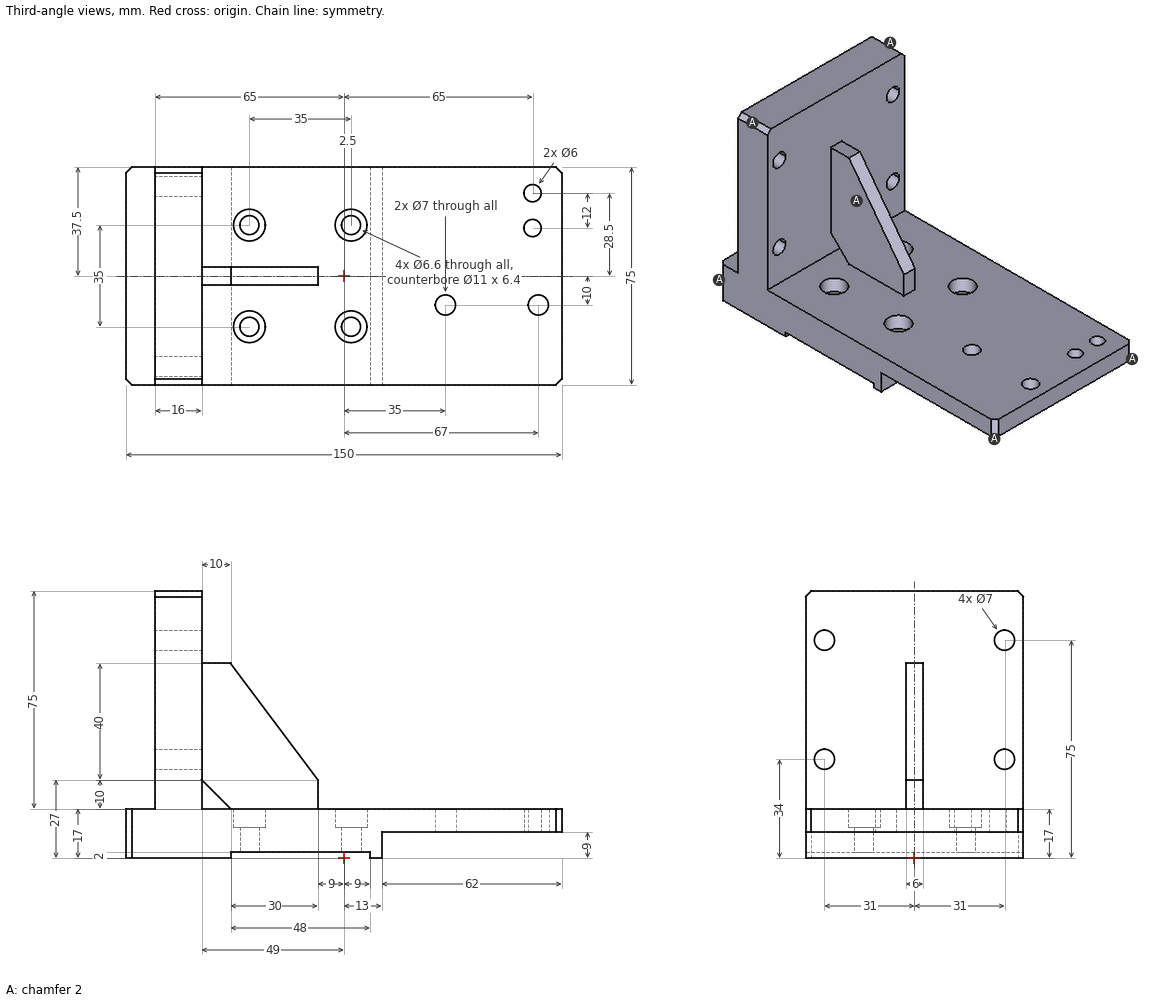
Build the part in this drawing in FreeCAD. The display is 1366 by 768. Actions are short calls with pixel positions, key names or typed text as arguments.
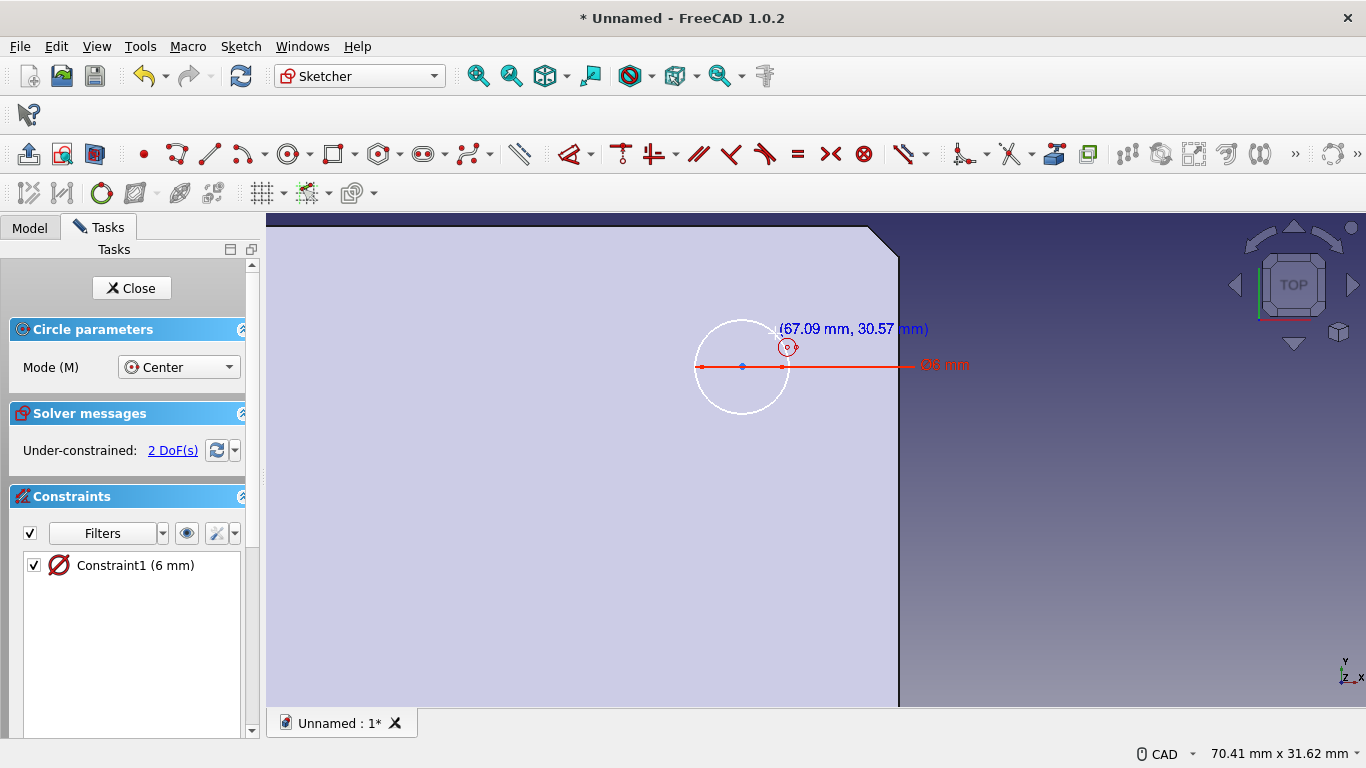
click(742, 554)
move(775, 521)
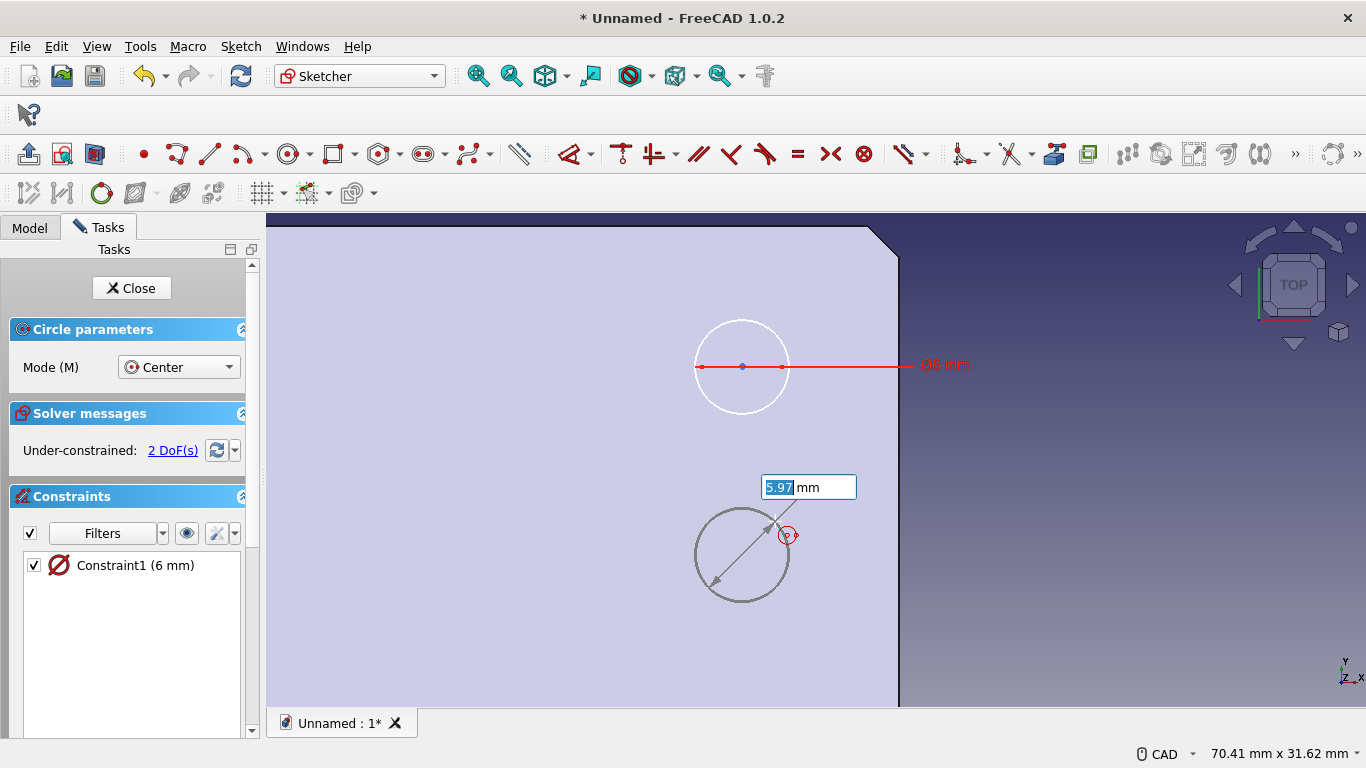
text(6)
key(Return)
key(Escape)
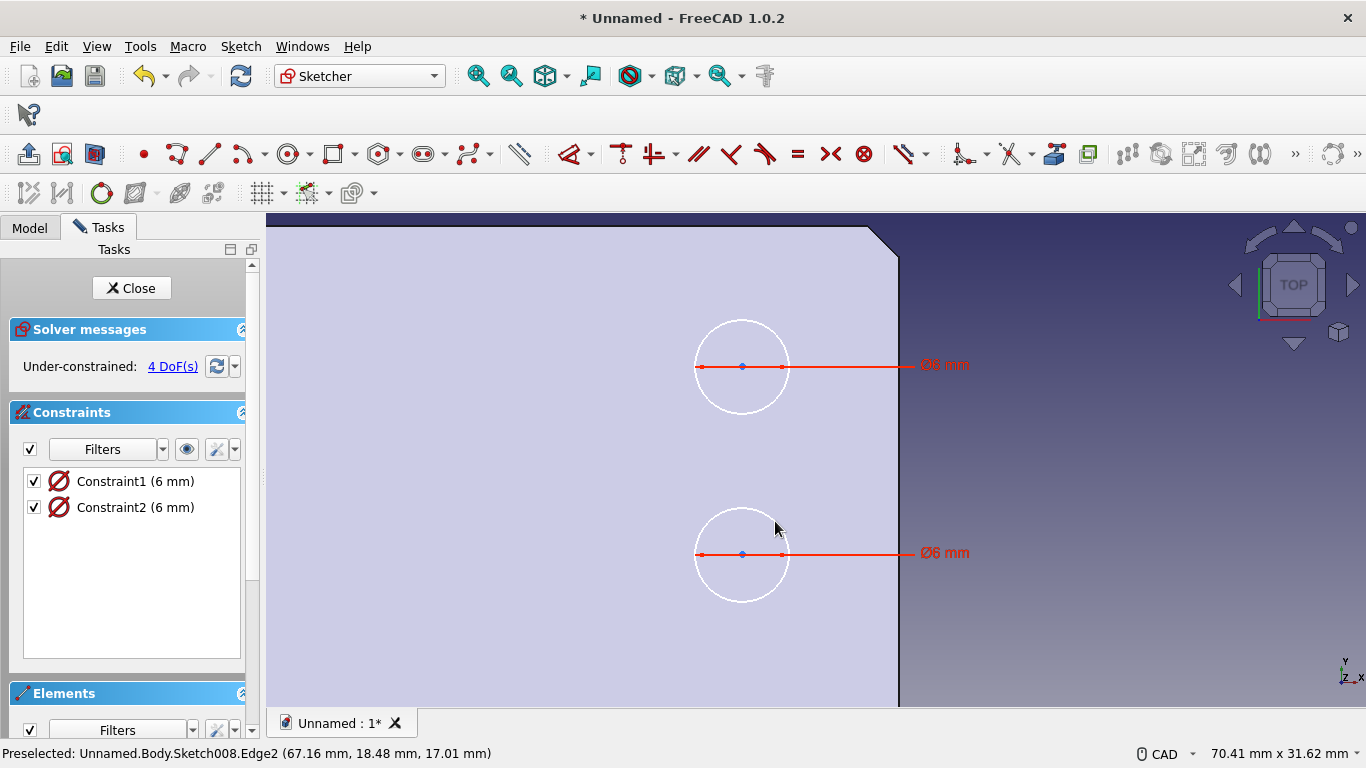
click(568, 154)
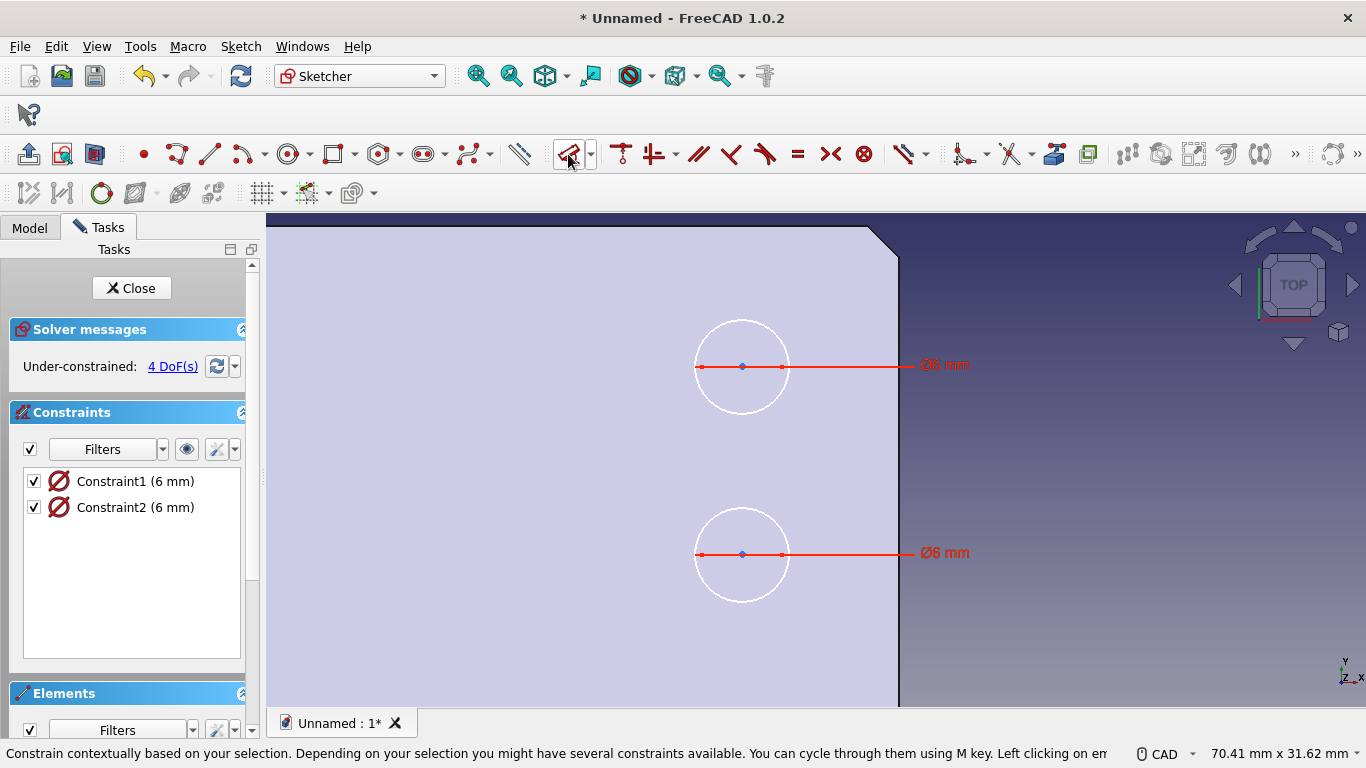
click(742, 367)
click(518, 333)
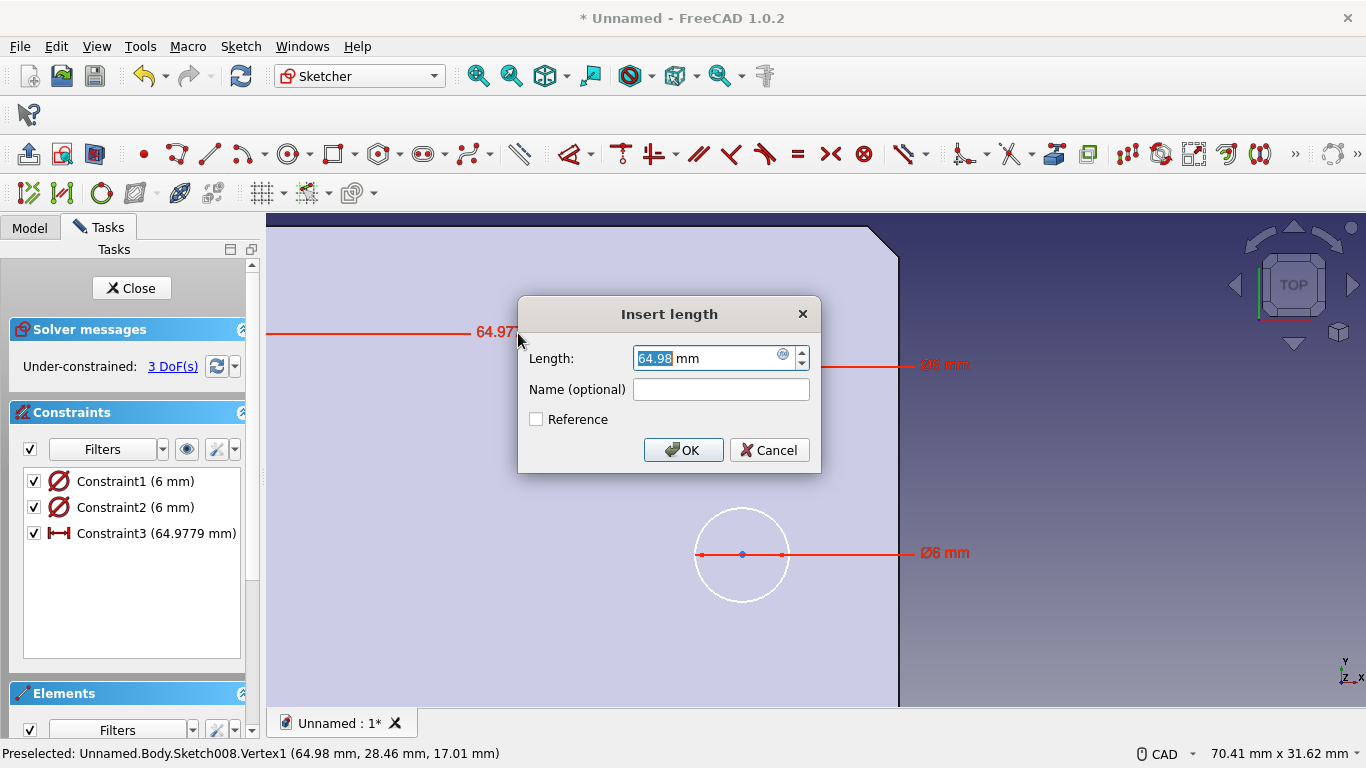
text(65)
key(Return)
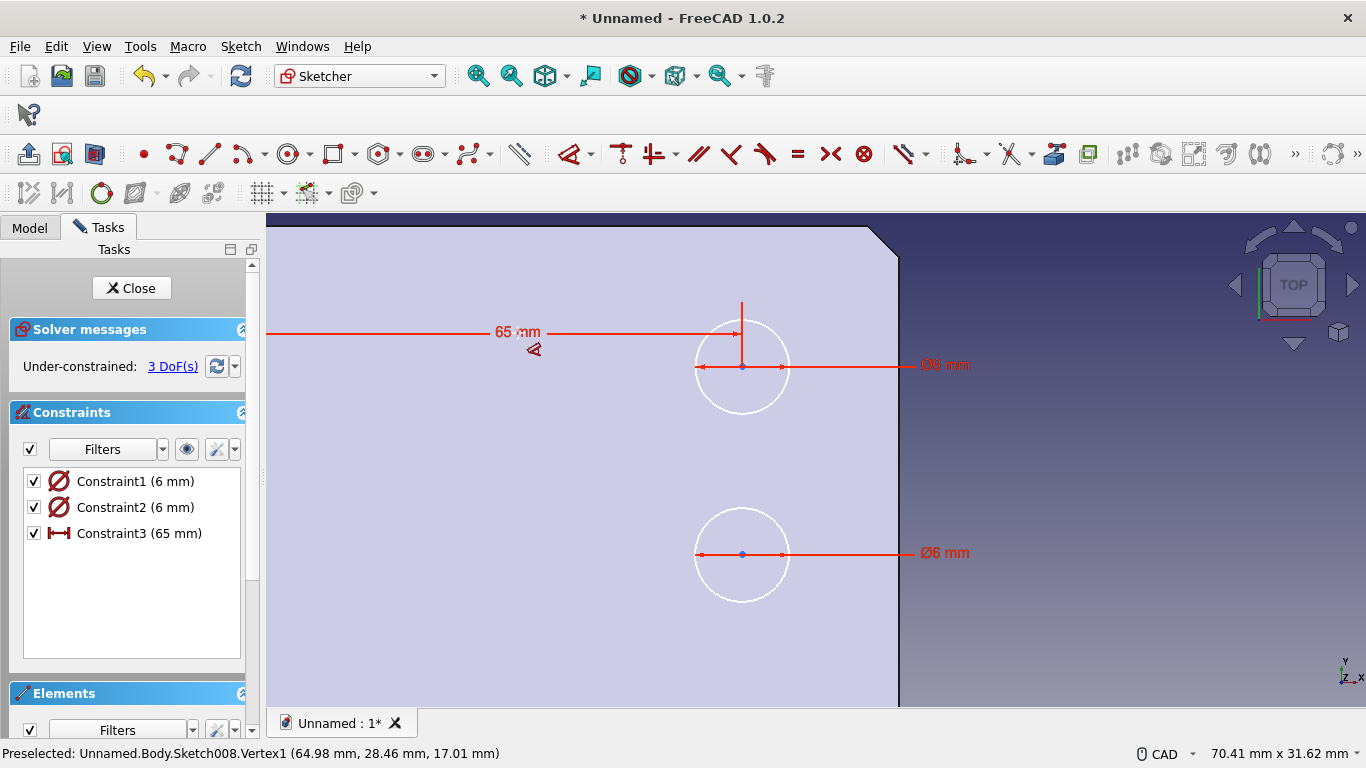
click(742, 555)
click(518, 521)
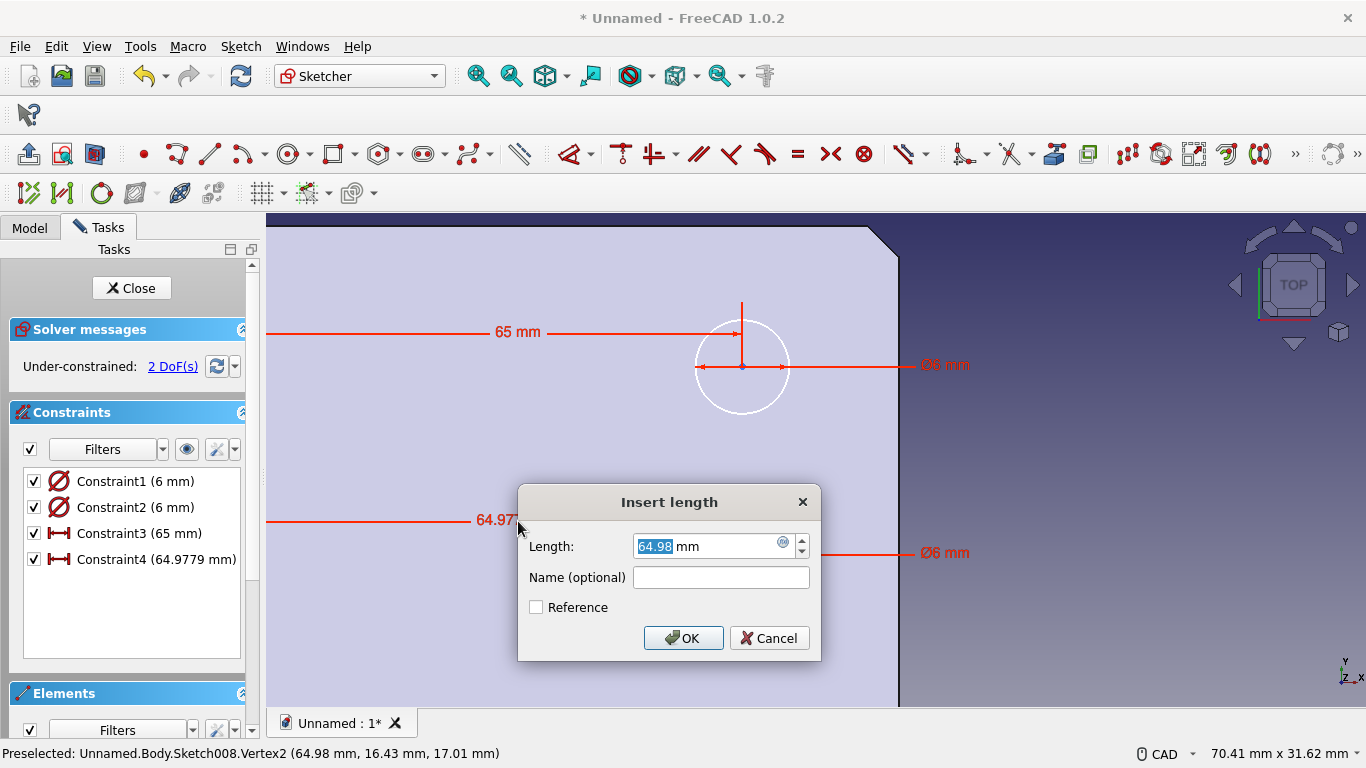
text(65)
key(Return)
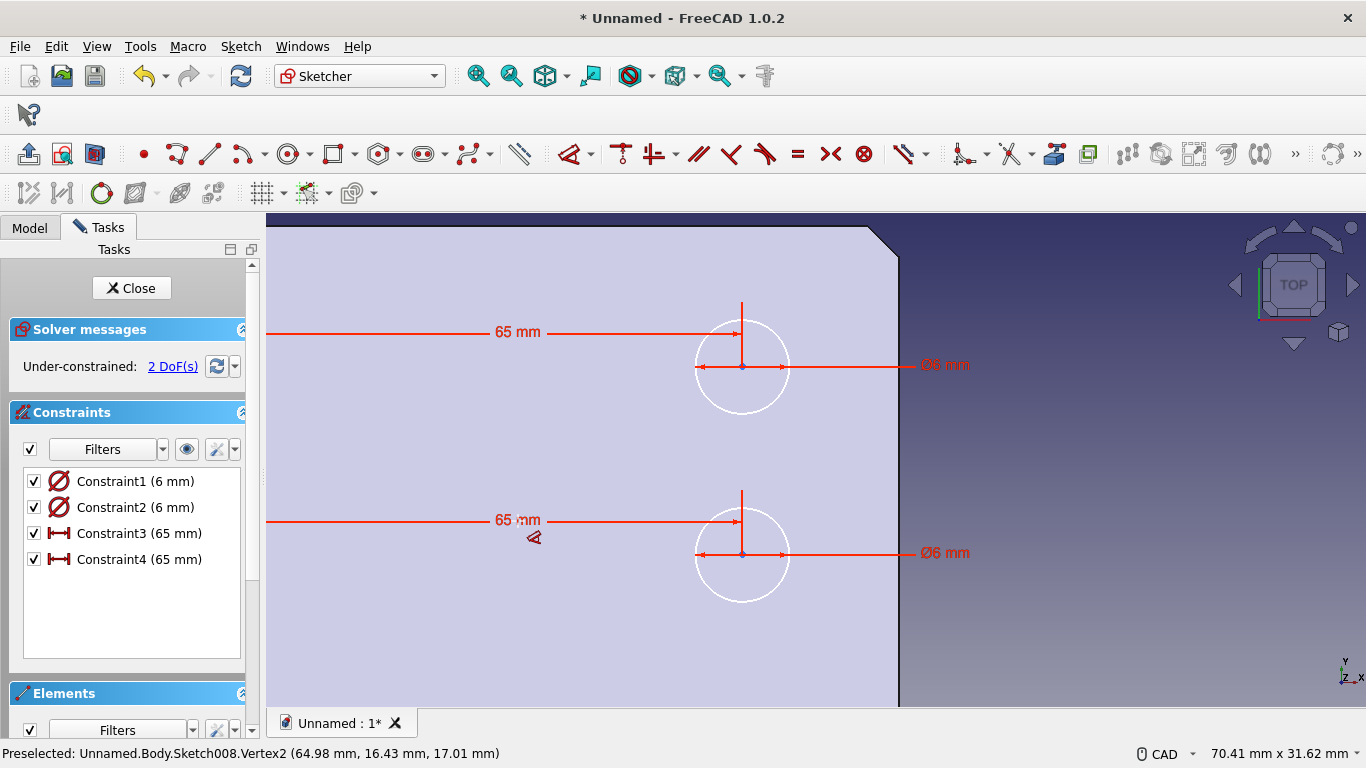
click(742, 367)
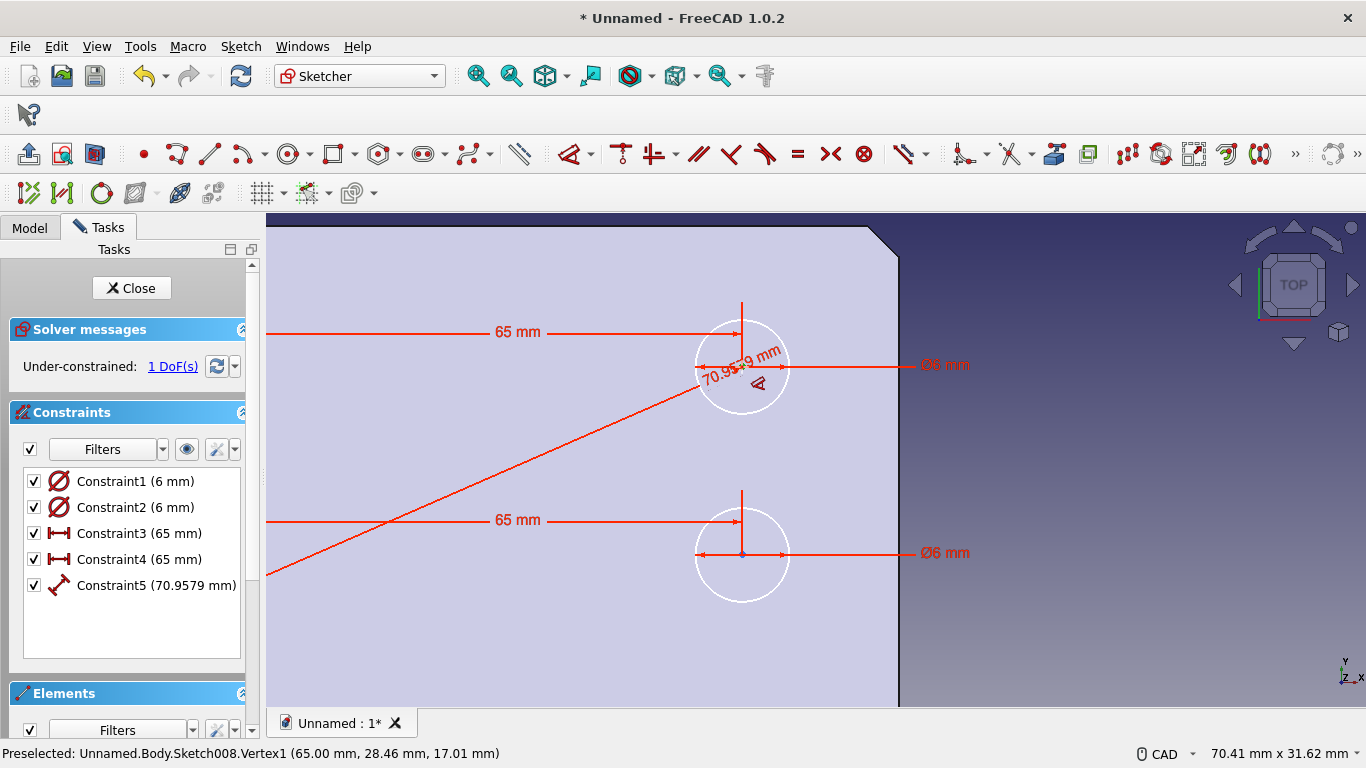
click(742, 555)
click(776, 461)